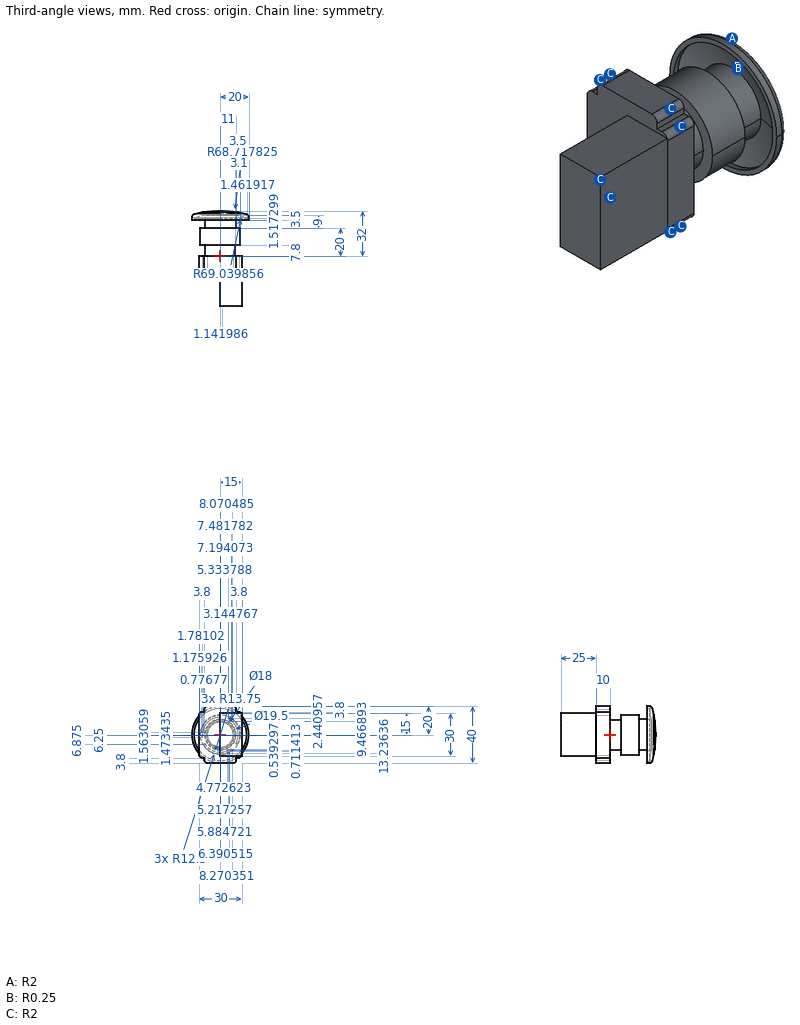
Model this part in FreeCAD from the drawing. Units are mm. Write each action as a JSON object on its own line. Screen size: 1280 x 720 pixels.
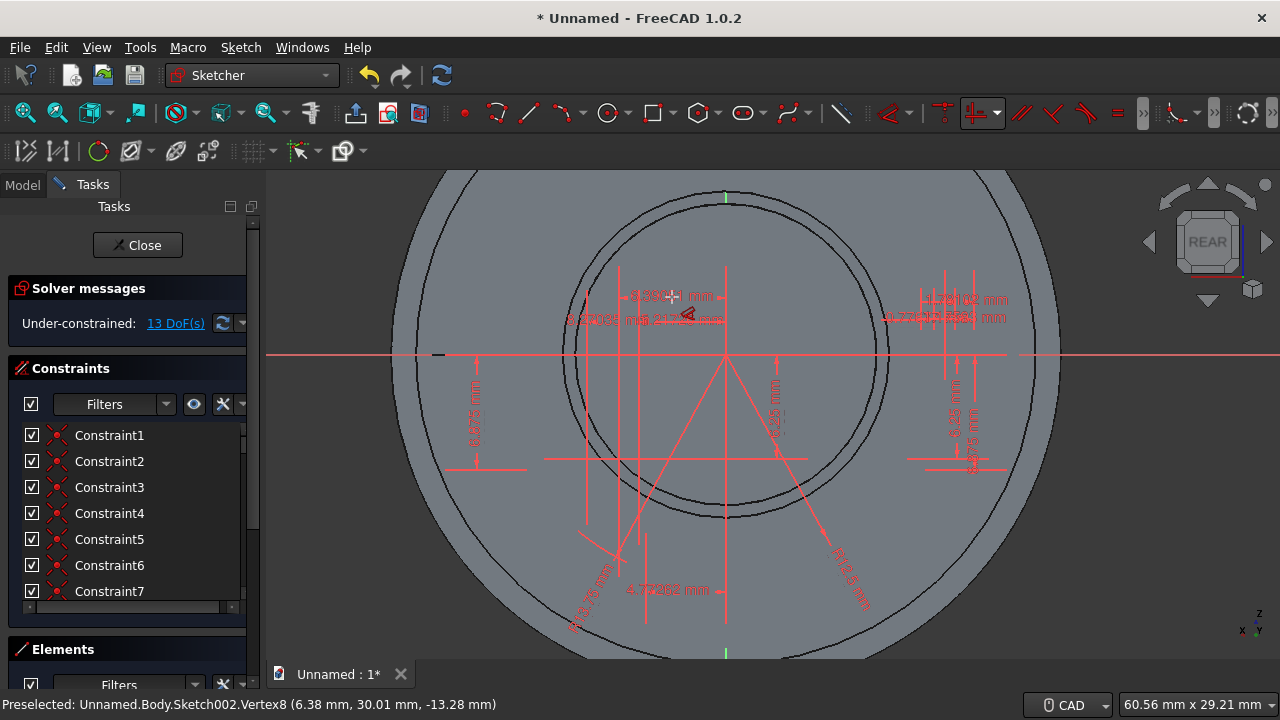
{"action": "left_click", "coordinate": [619, 577]}
{"action": "left_click", "coordinate": [585, 466]}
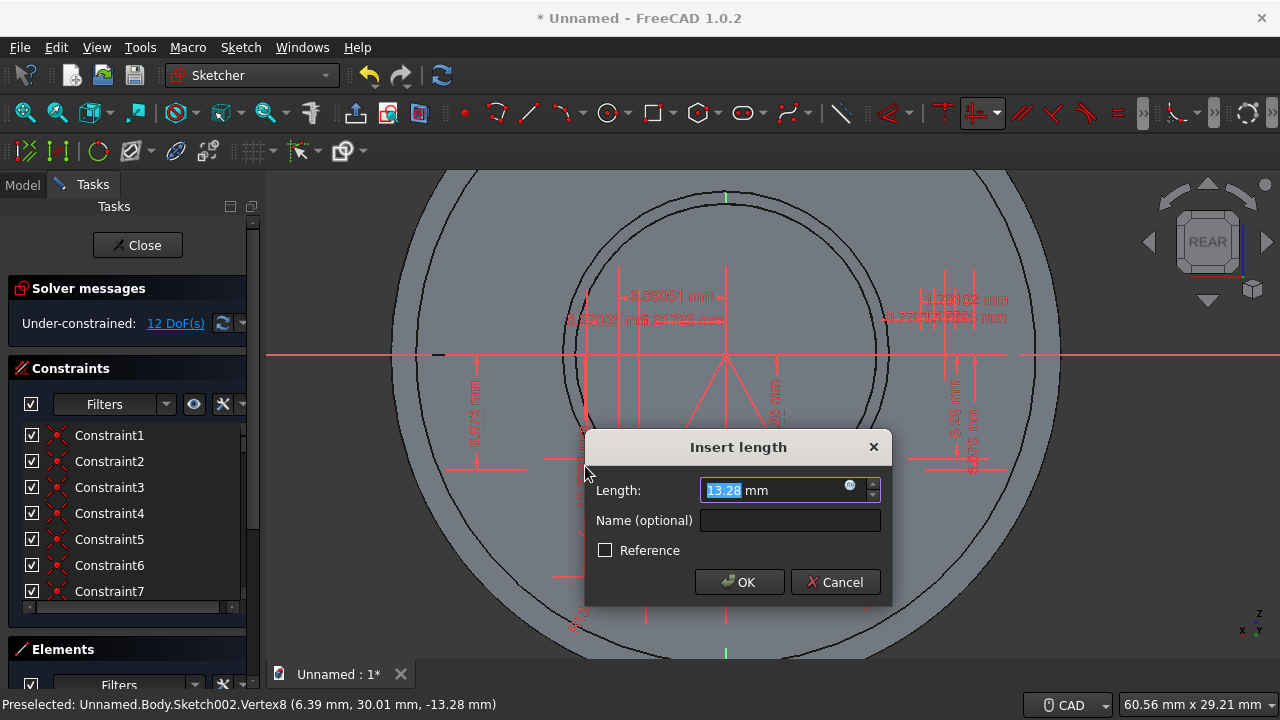
{"action": "type", "text": "13.23636"}
{"action": "key", "text": "Return"}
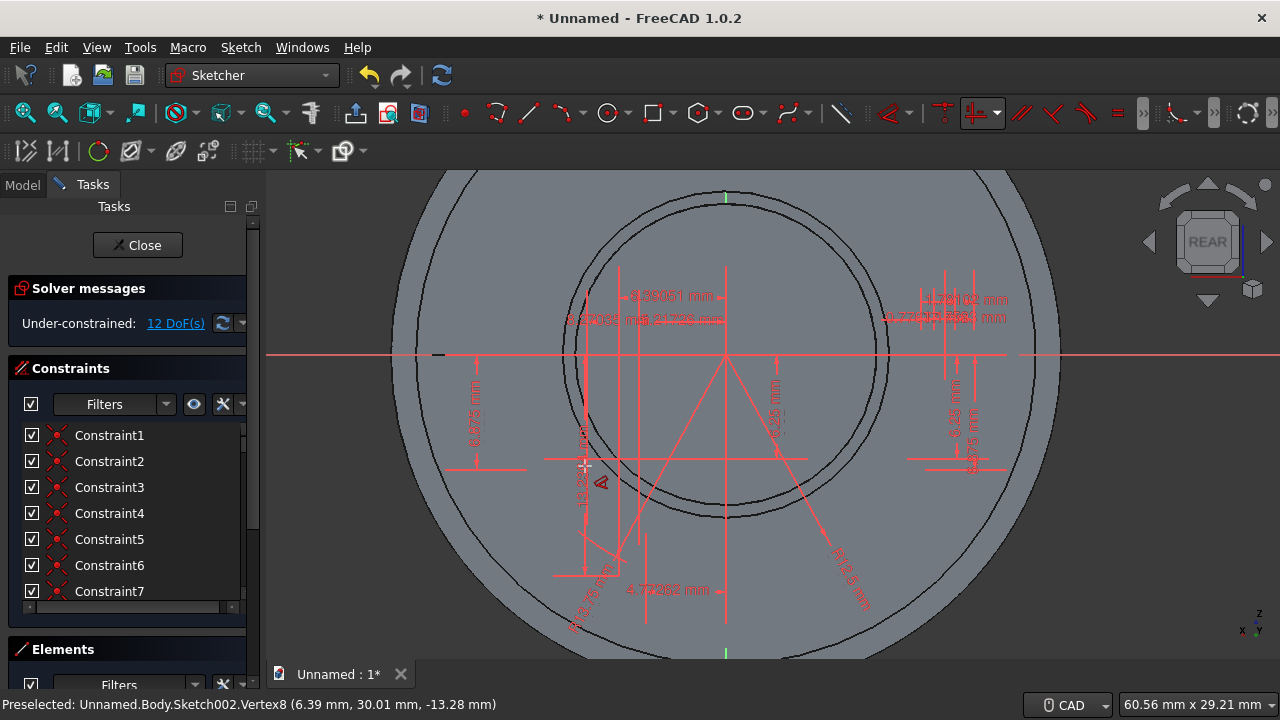
{"action": "left_click", "coordinate": [627, 563]}
{"action": "left_click", "coordinate": [677, 621]}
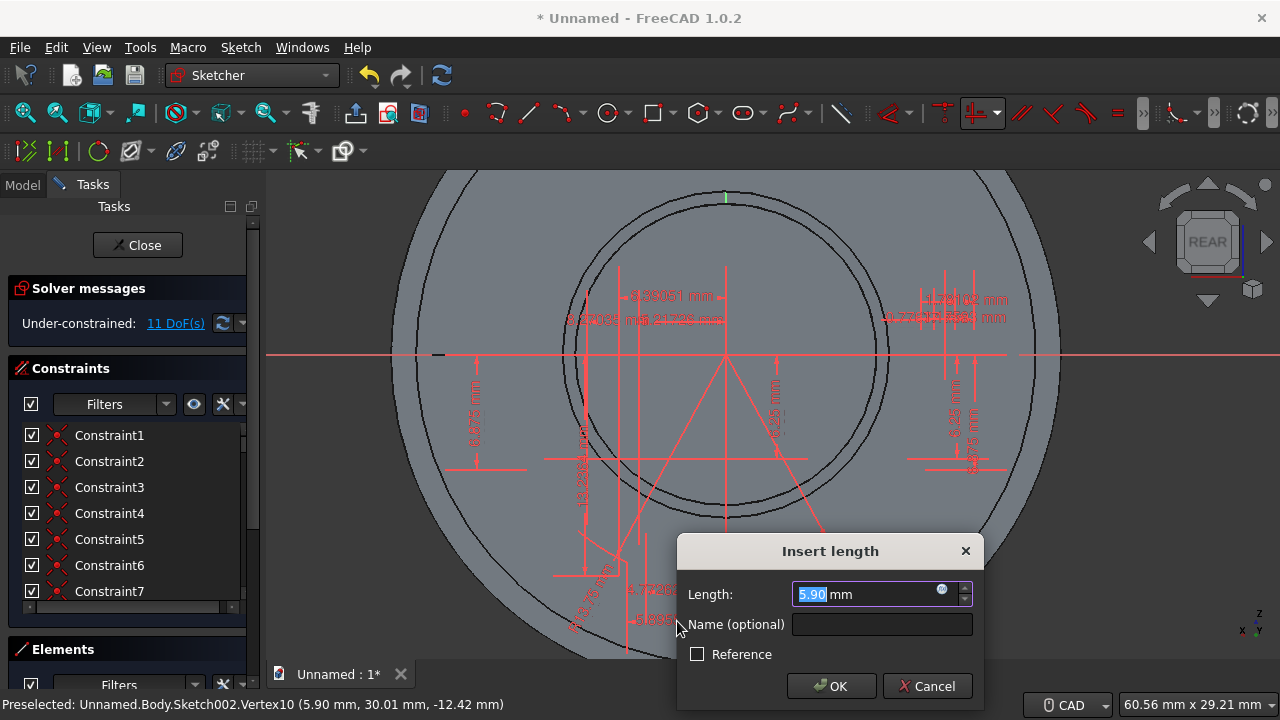
{"action": "type", "text": "5.884721"}
{"action": "key", "text": "Return"}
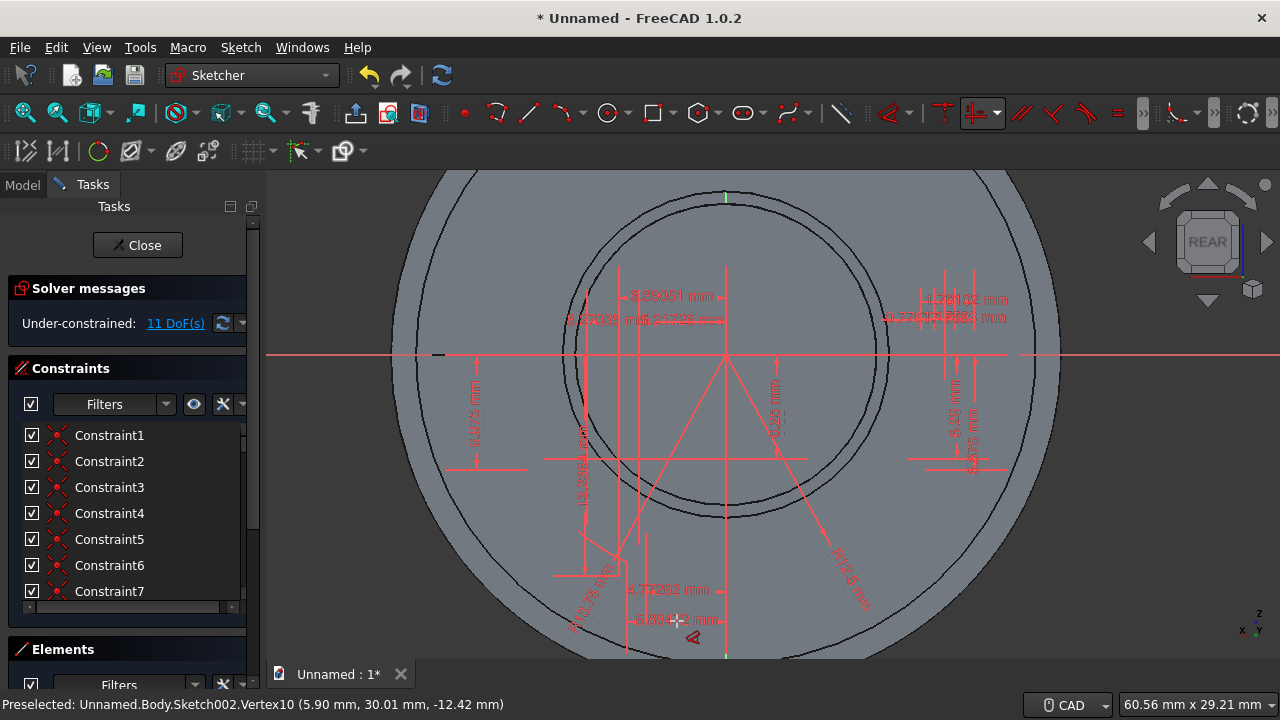
{"action": "scroll", "coordinate": [934, 330], "scroll_direction": "up", "scroll_amount": 3}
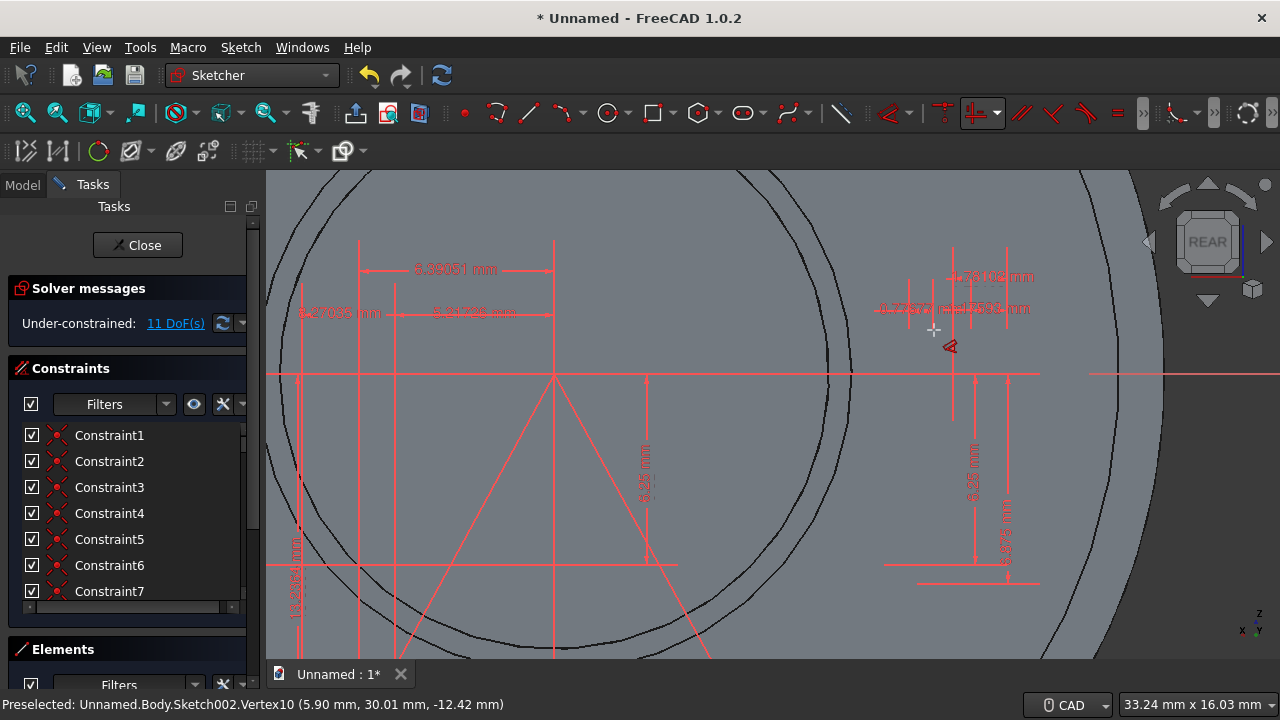
{"action": "left_click", "coordinate": [933, 329]}
{"action": "left_click", "coordinate": [967, 352]}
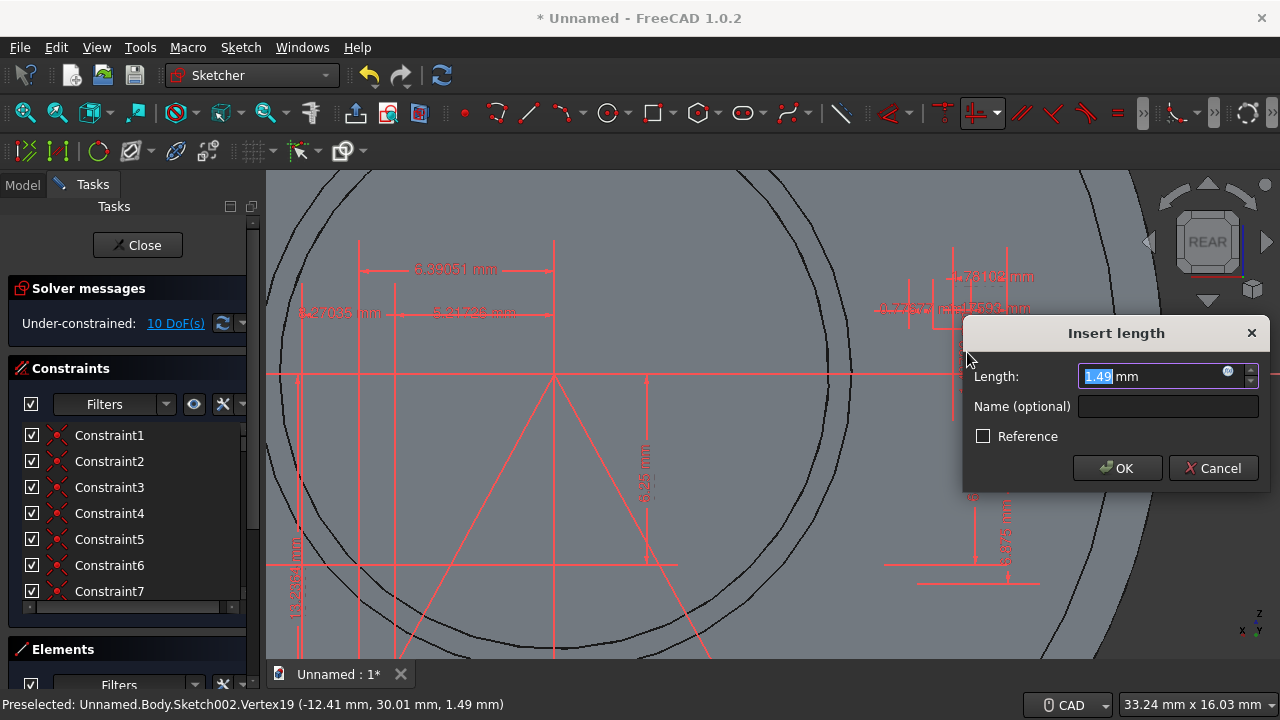
{"action": "type", "text": "1.563059"}
{"action": "key", "text": "Return"}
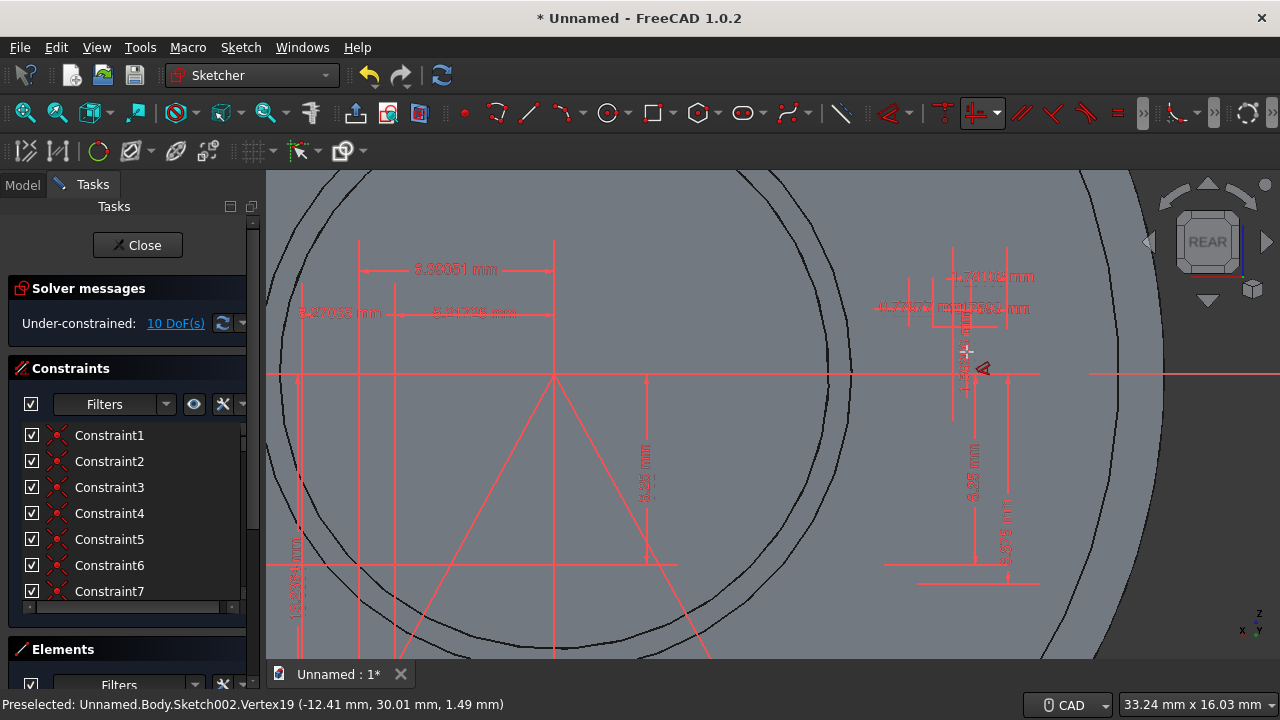
{"action": "left_click", "coordinate": [953, 421]}
{"action": "left_click", "coordinate": [987, 398]}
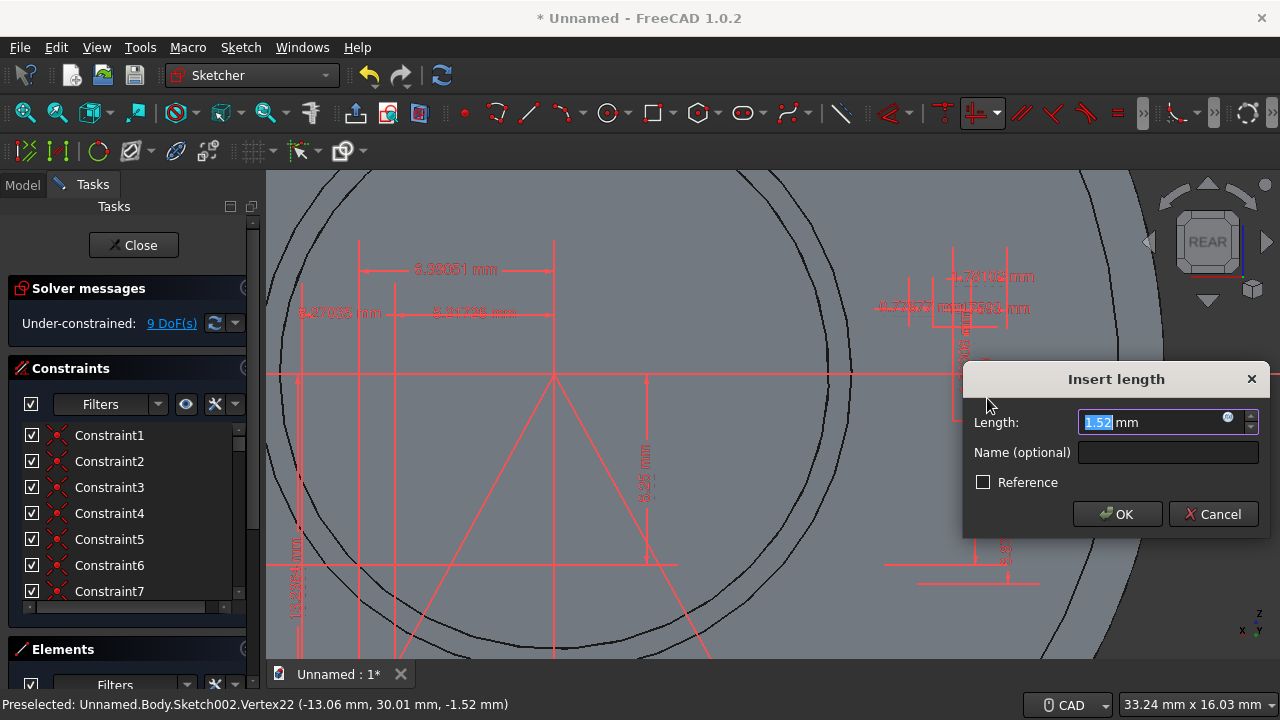
{"action": "type", "text": "1.473435"}
{"action": "key", "text": "Return"}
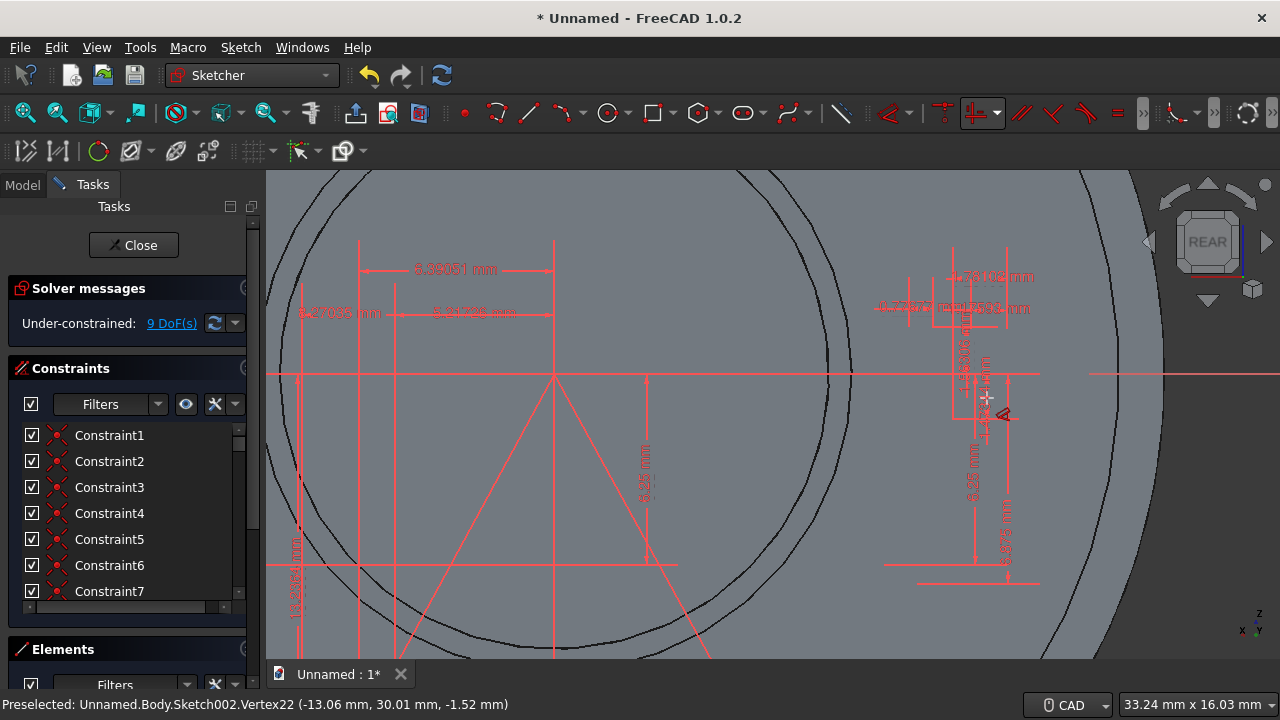
{"action": "left_click", "coordinate": [1007, 328]}
{"action": "left_click", "coordinate": [1041, 351]}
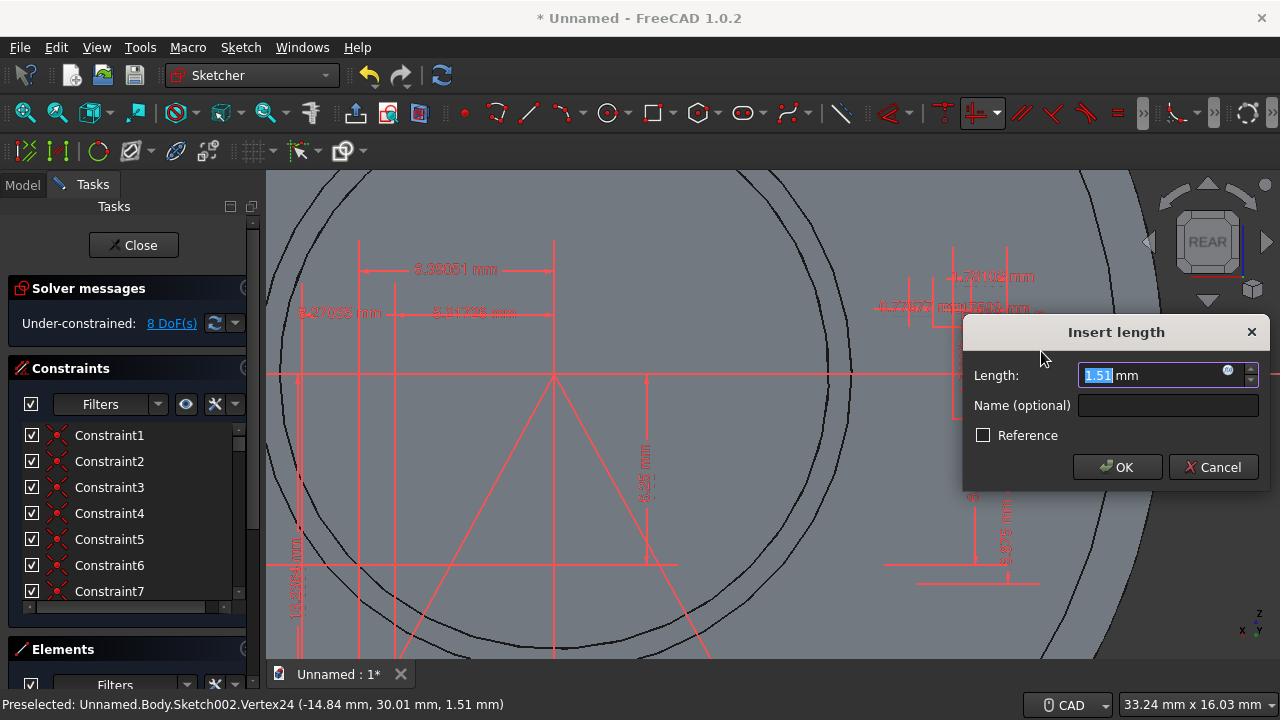
{"action": "type", "text": "1.563059"}
{"action": "key", "text": "Return"}